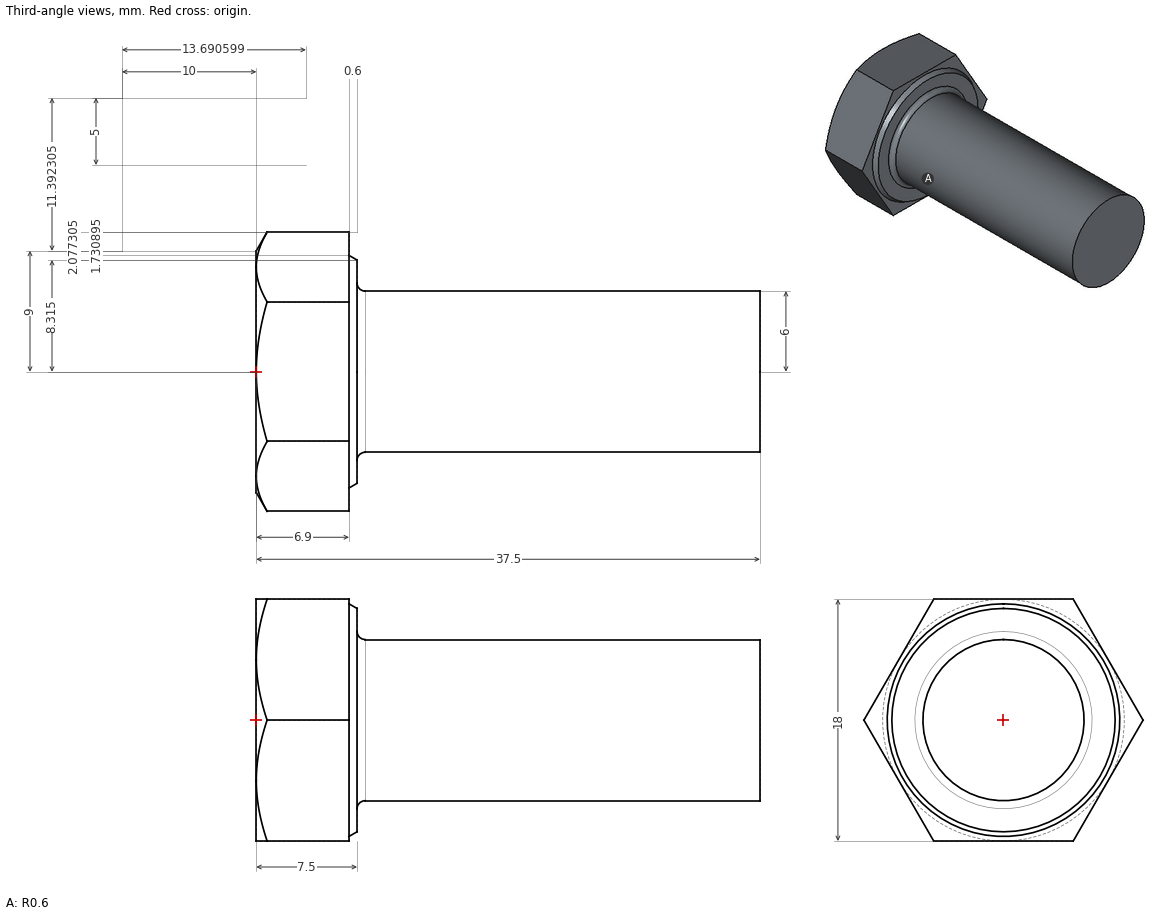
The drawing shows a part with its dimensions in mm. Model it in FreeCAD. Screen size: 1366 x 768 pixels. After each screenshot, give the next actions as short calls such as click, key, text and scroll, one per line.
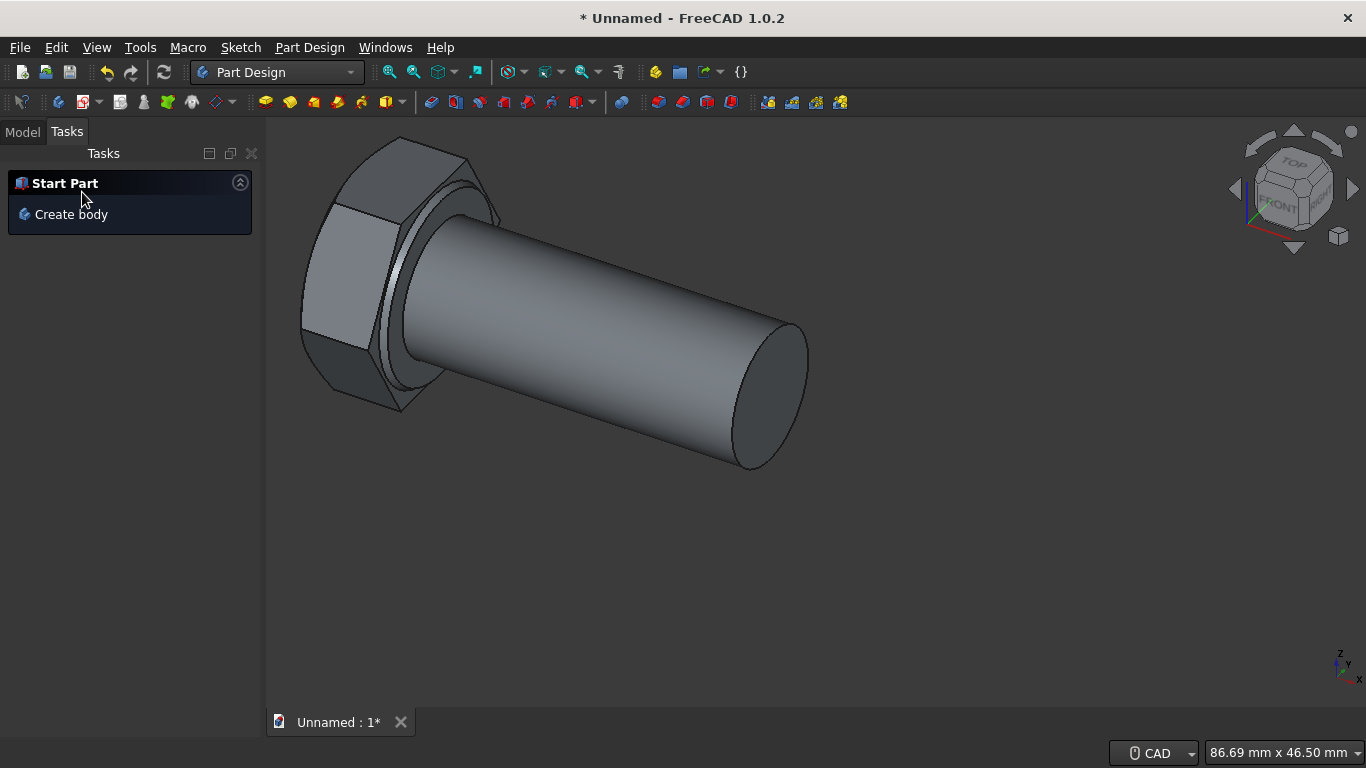
key(v)
key(f)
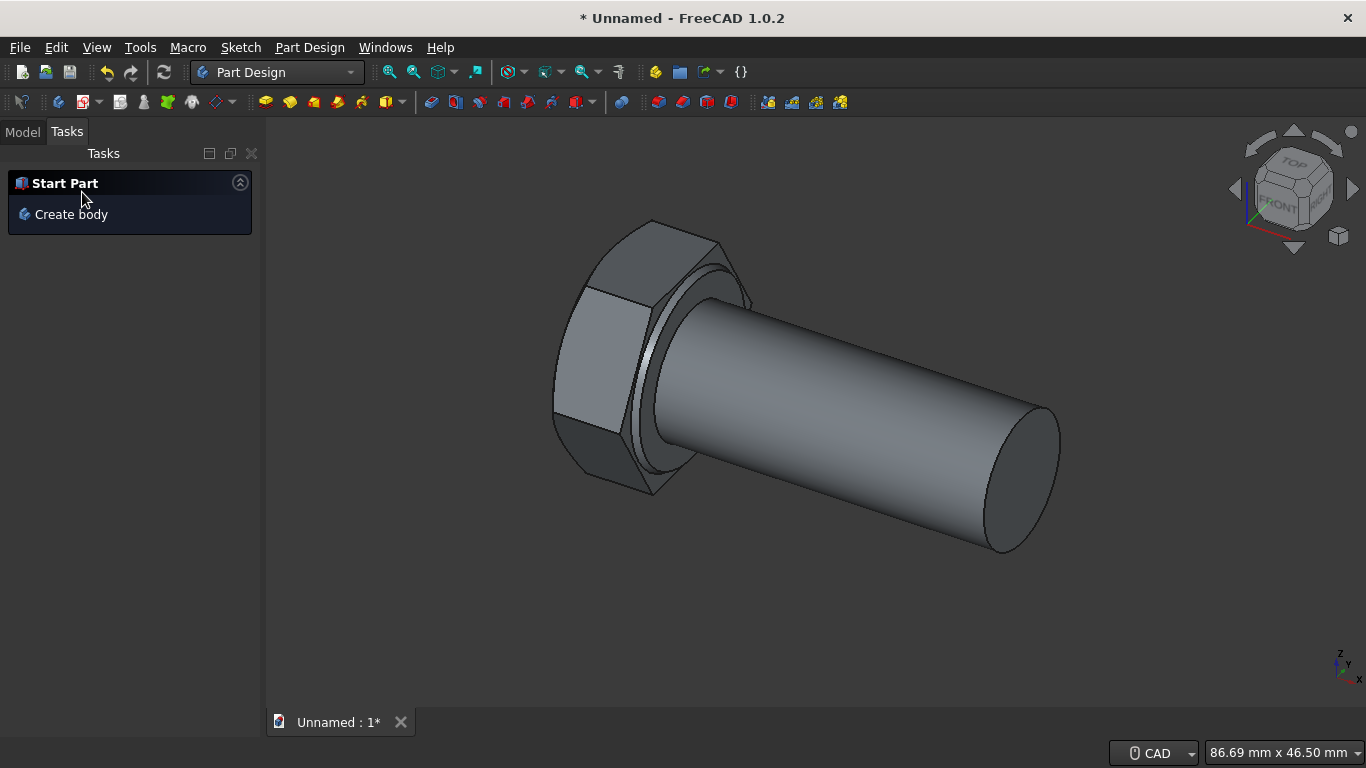
key(0)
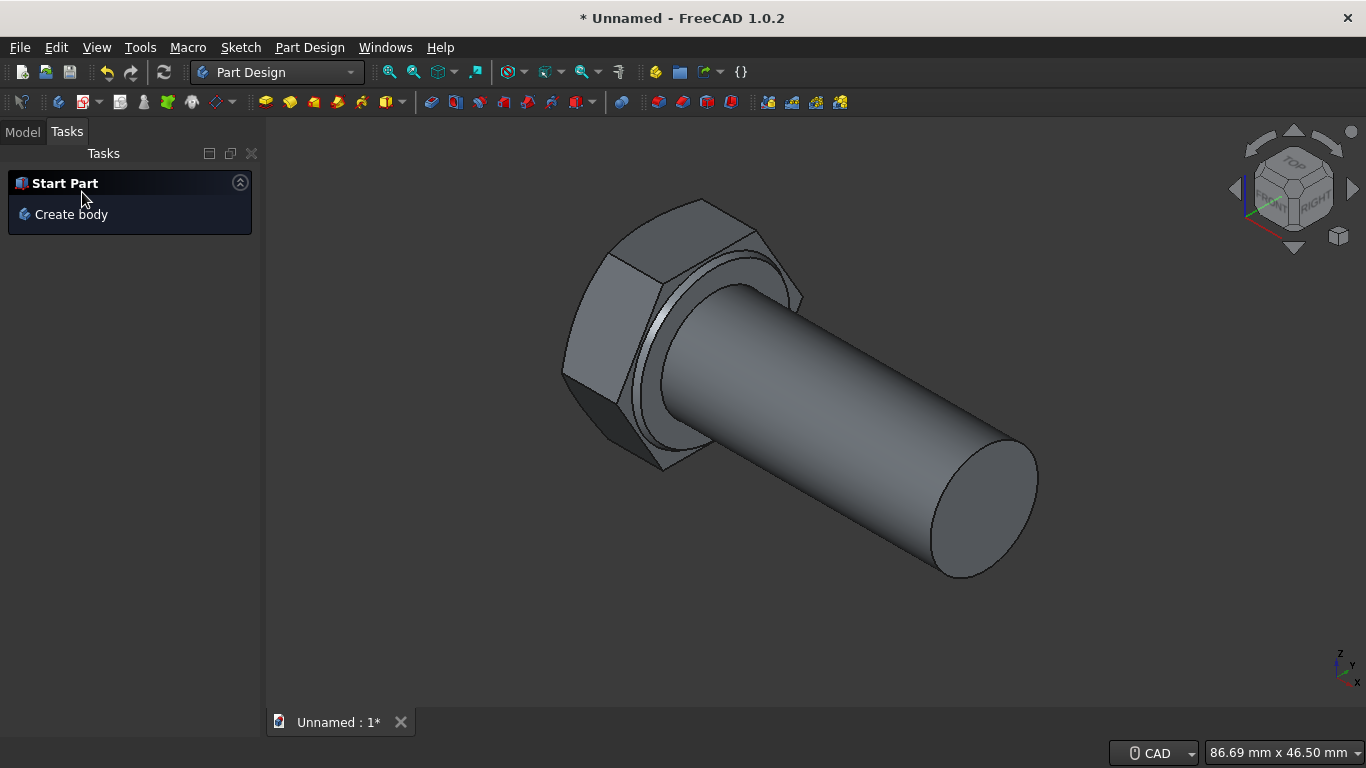
key(2)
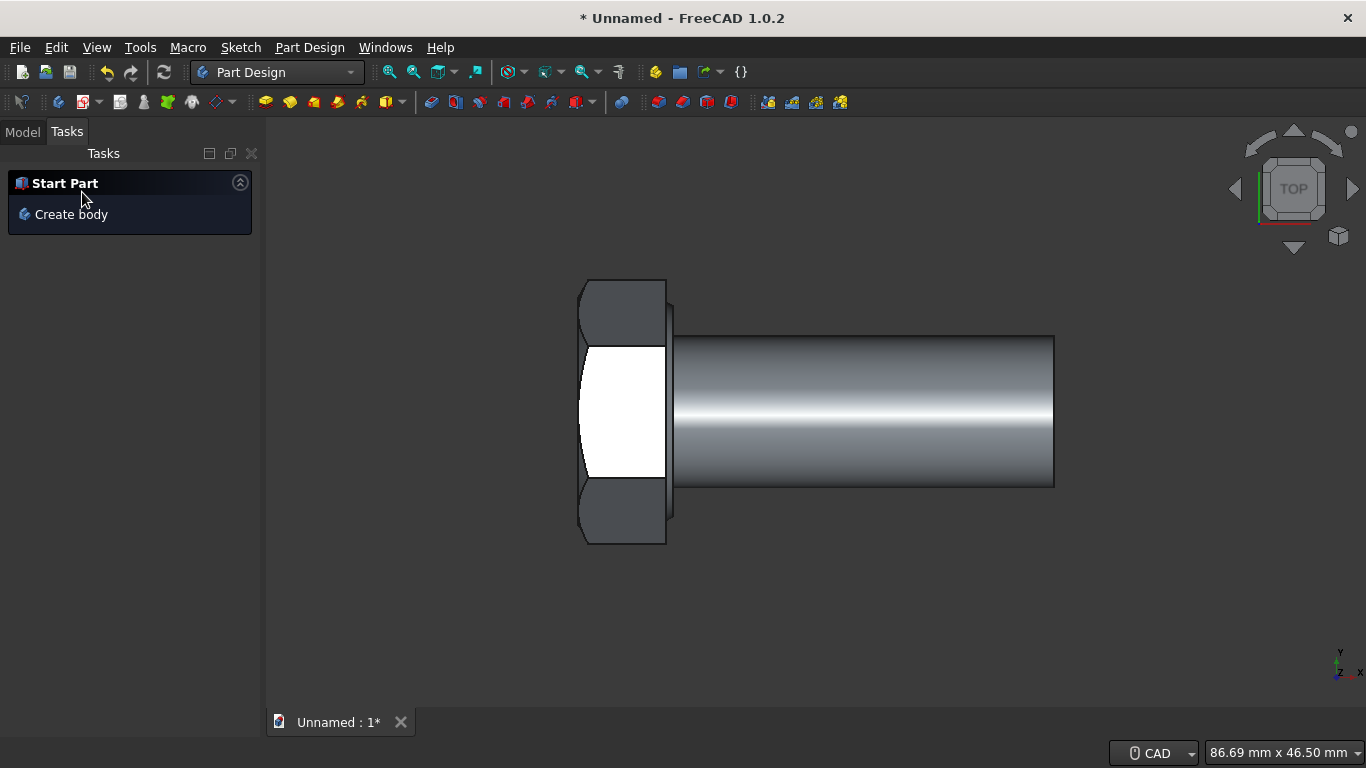
key(v)
key(f)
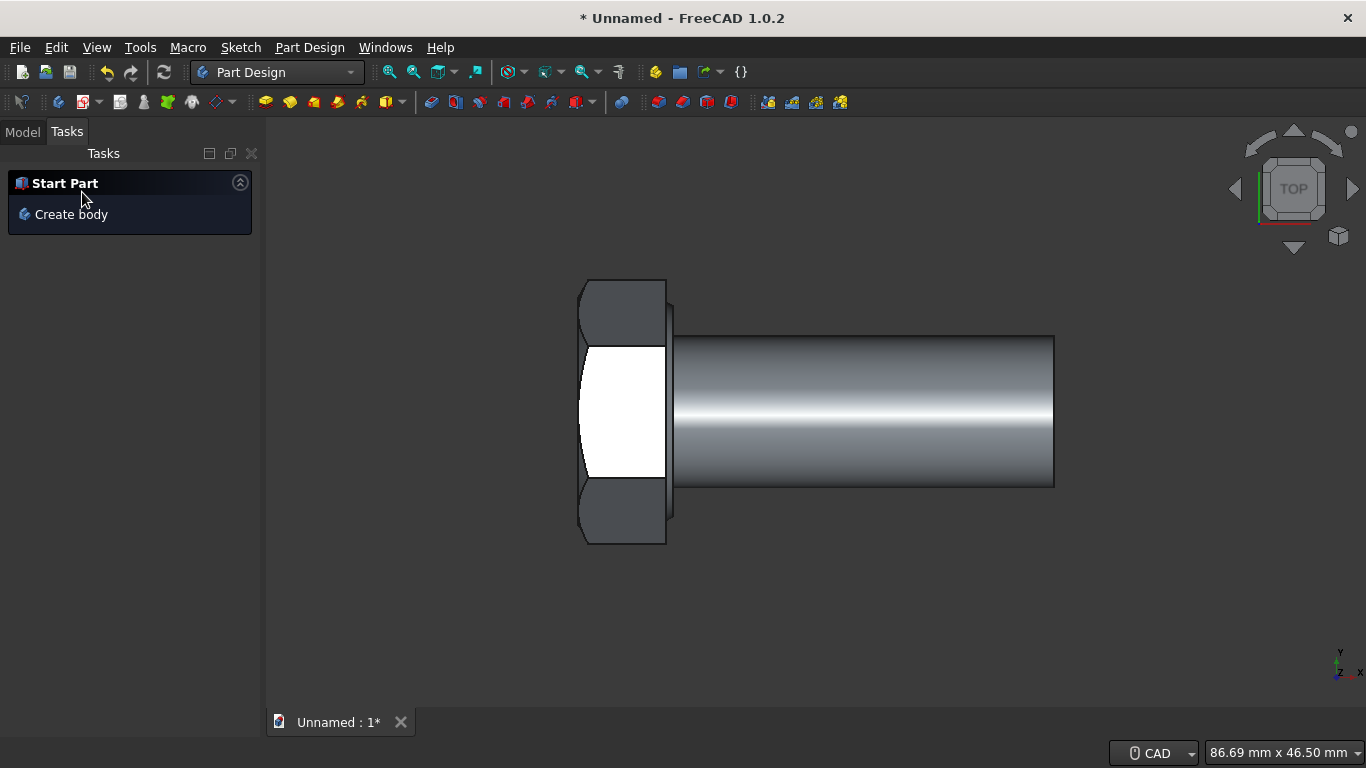
key(1)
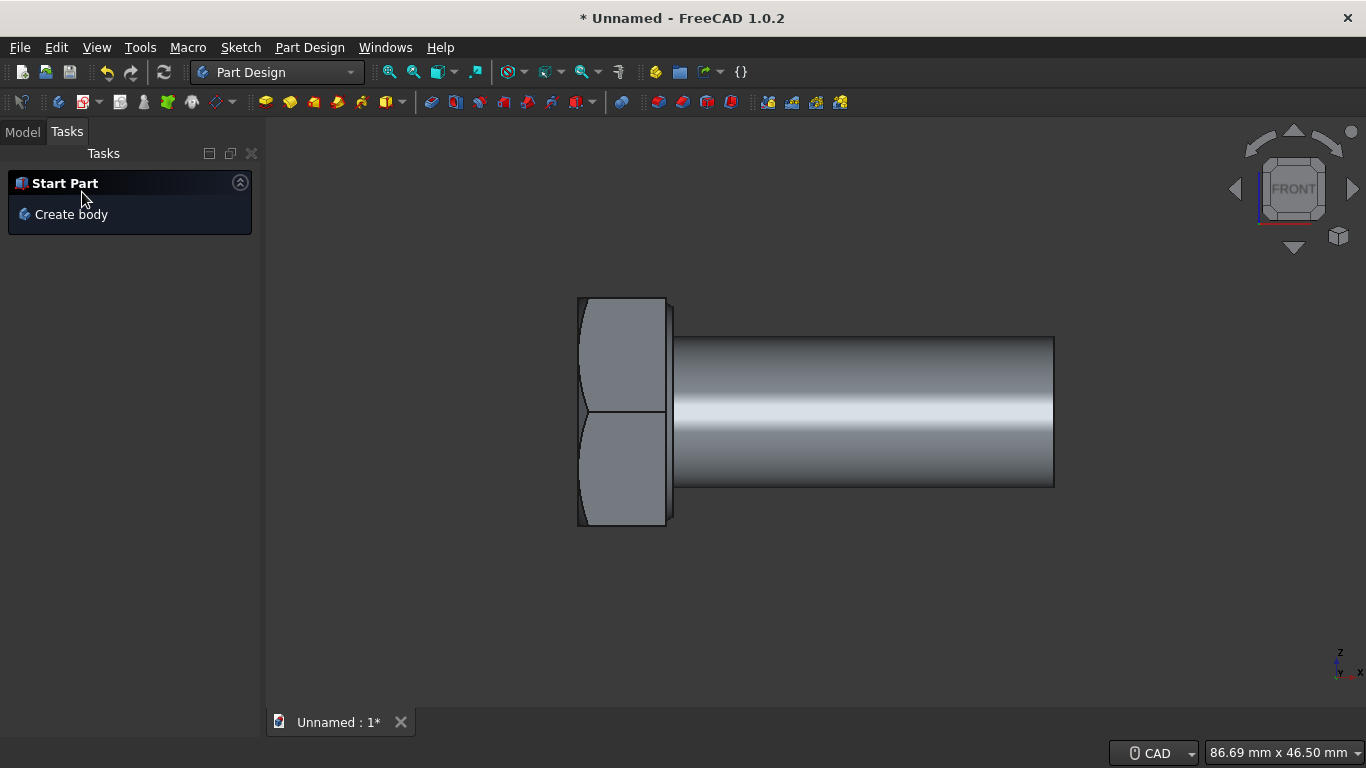
key(v)
key(f)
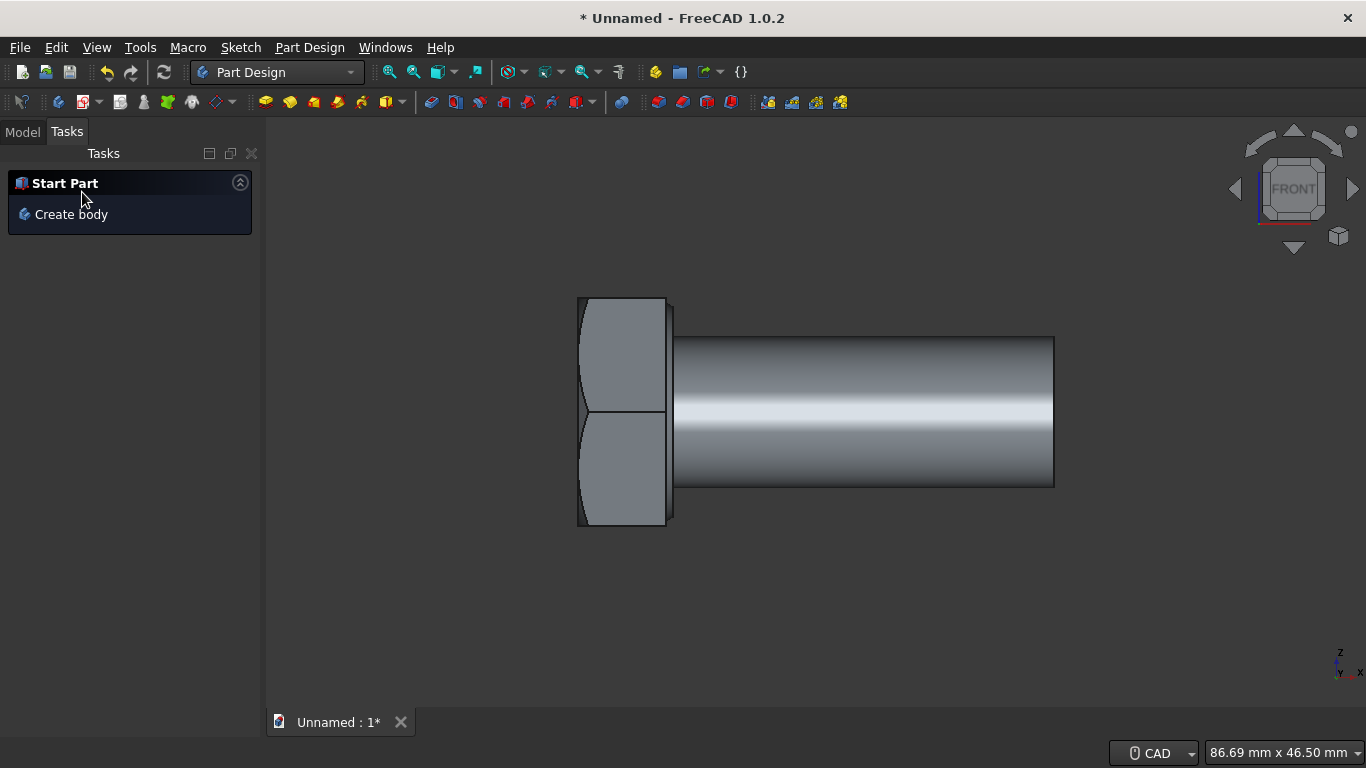
key(3)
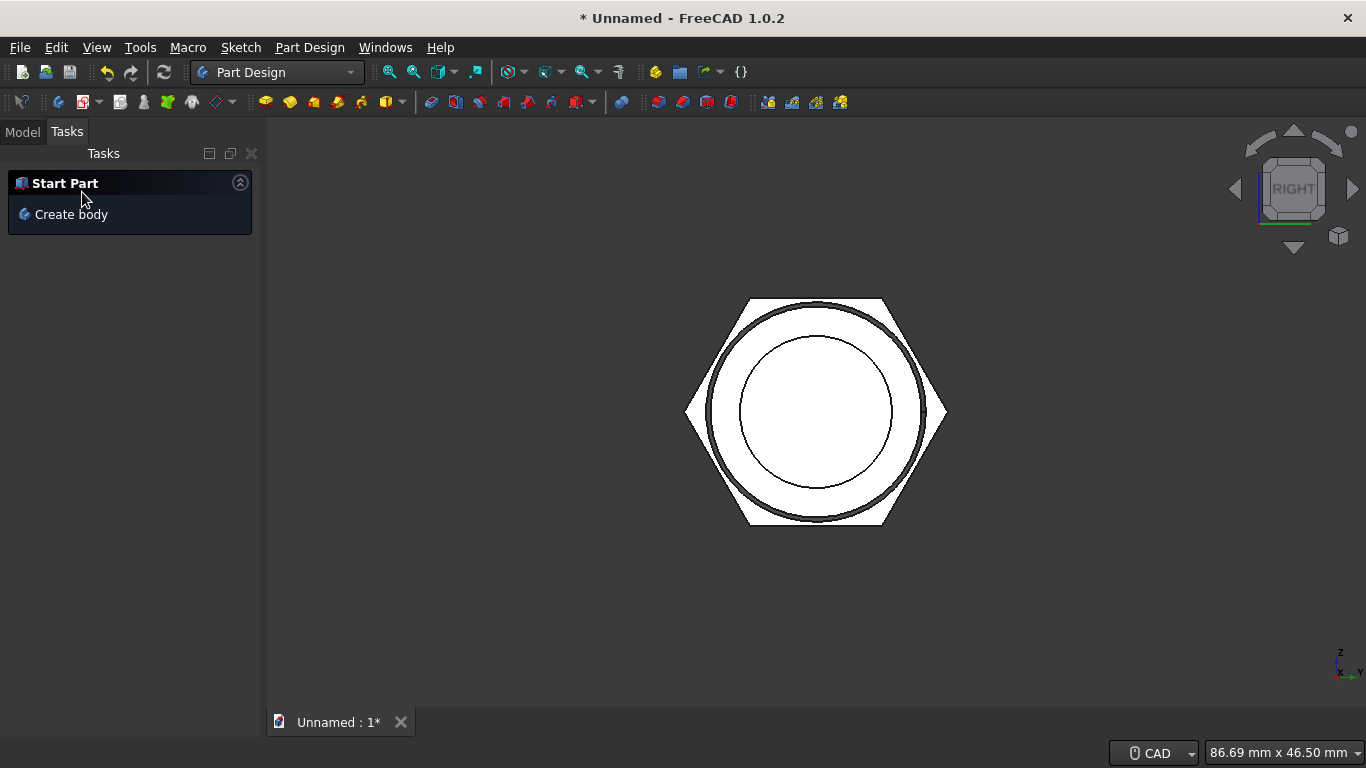
click(390, 72)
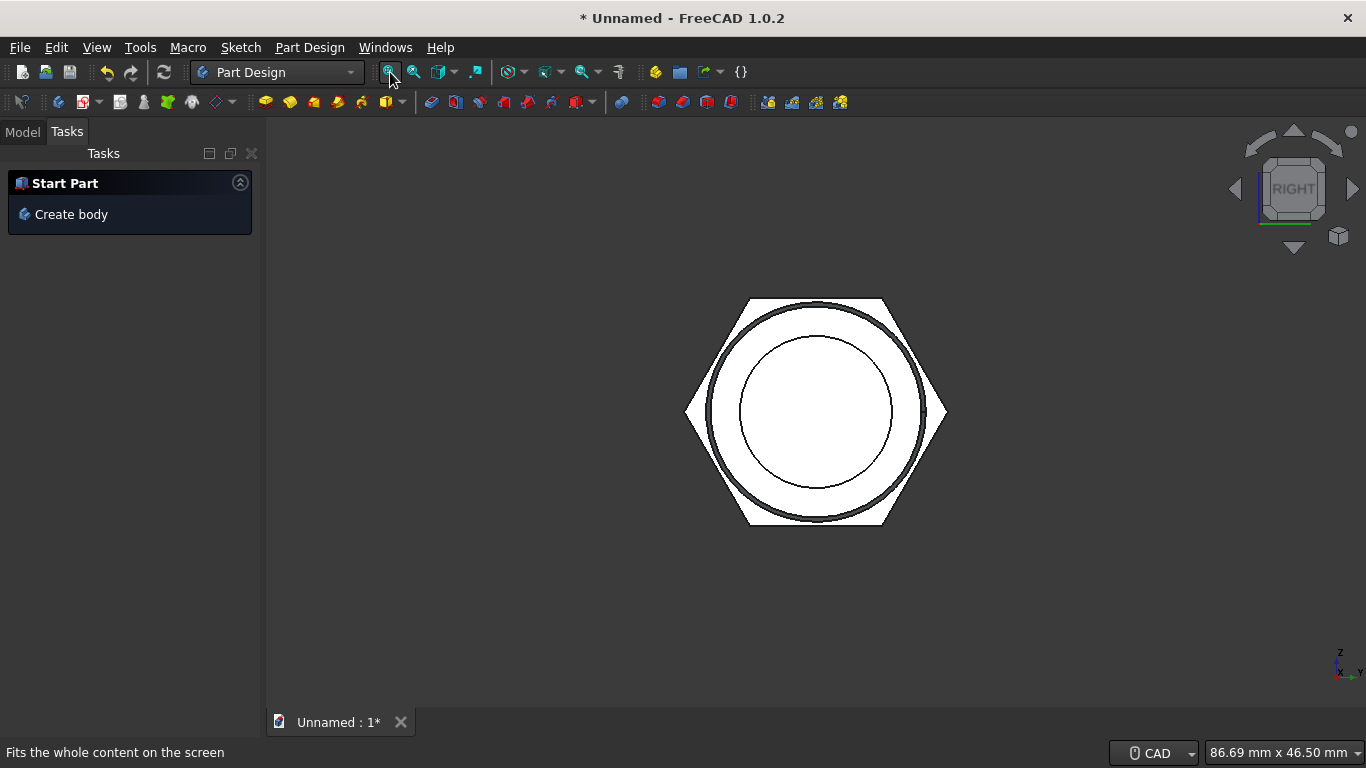
key(5)